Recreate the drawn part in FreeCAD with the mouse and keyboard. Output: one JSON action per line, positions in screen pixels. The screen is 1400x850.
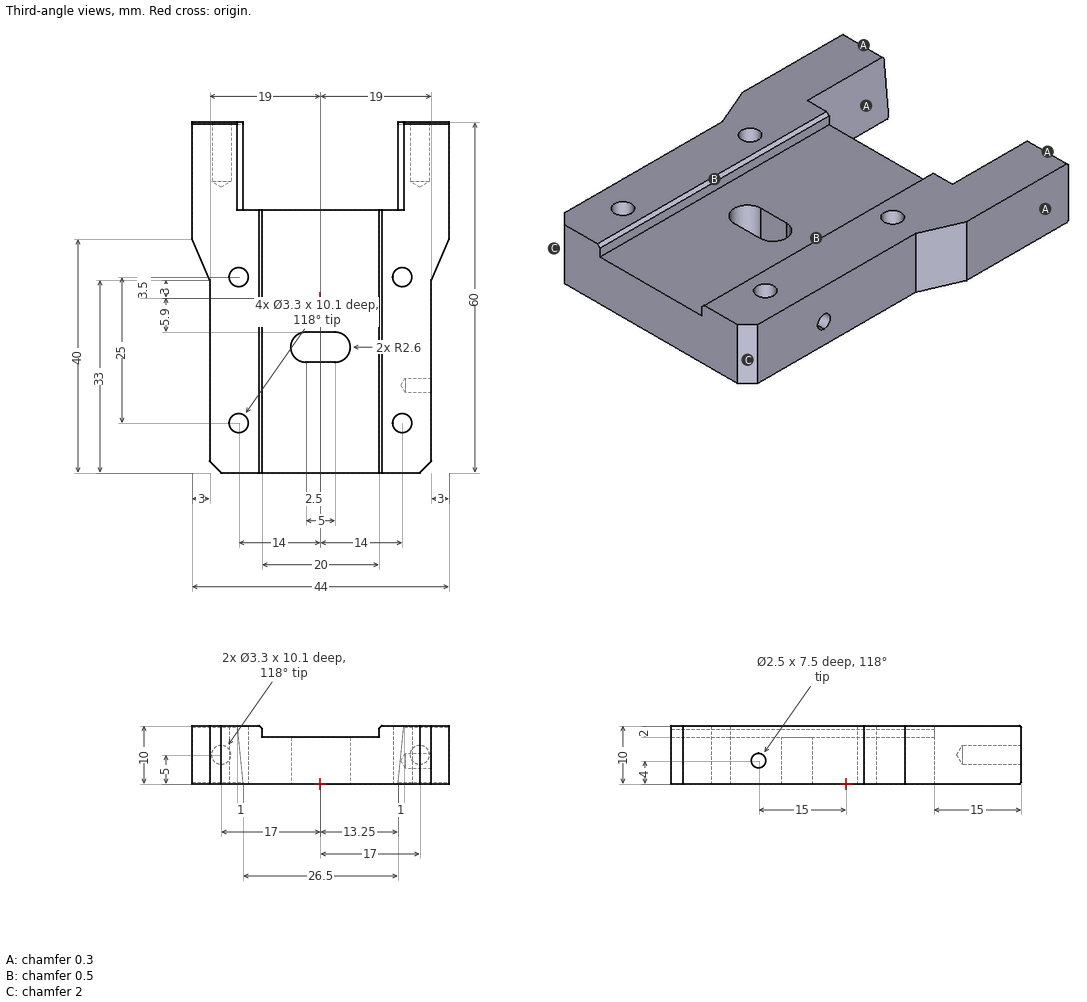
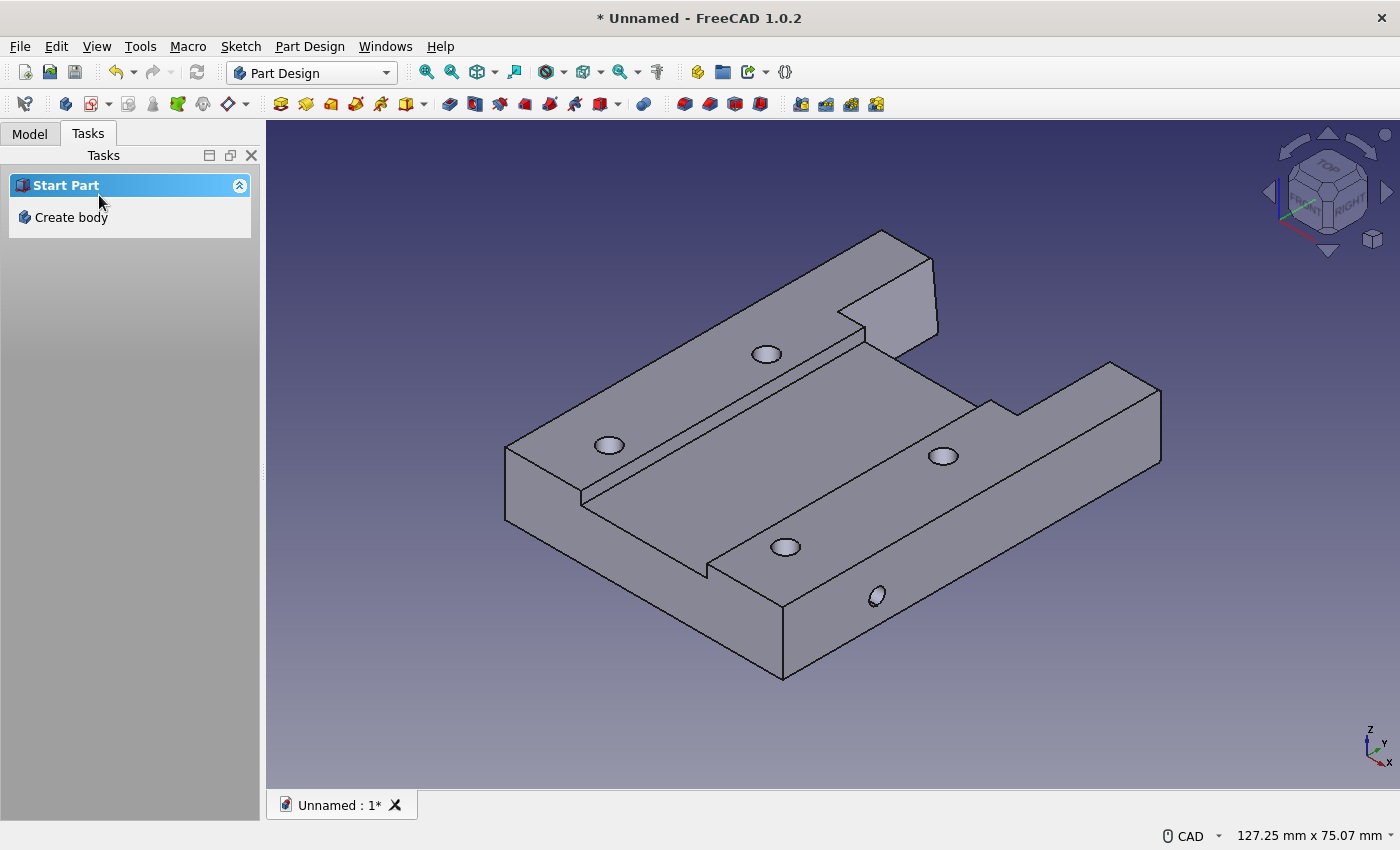
{"action": "left_click", "coordinate": [723, 408]}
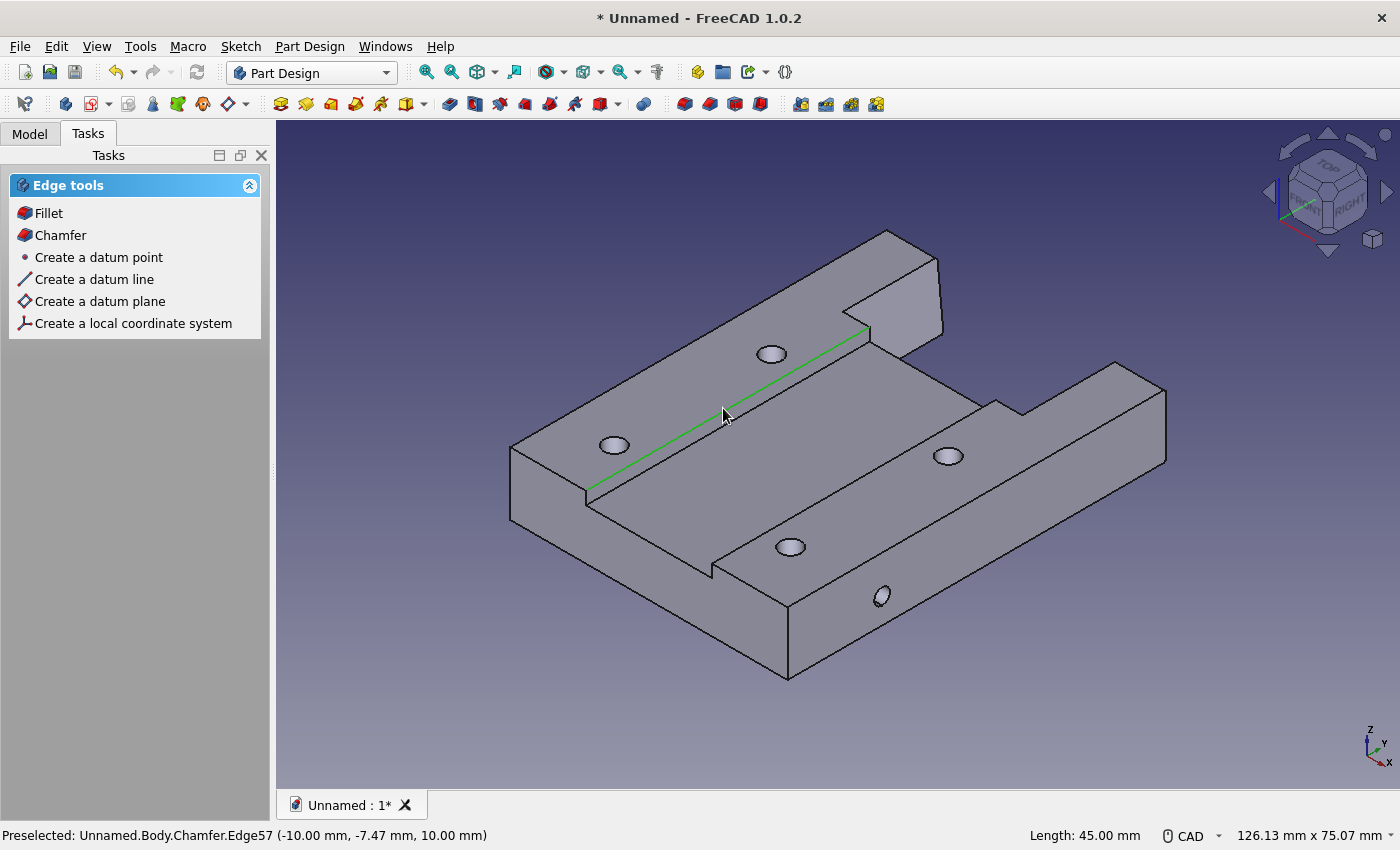
{"action": "key", "text": "2"}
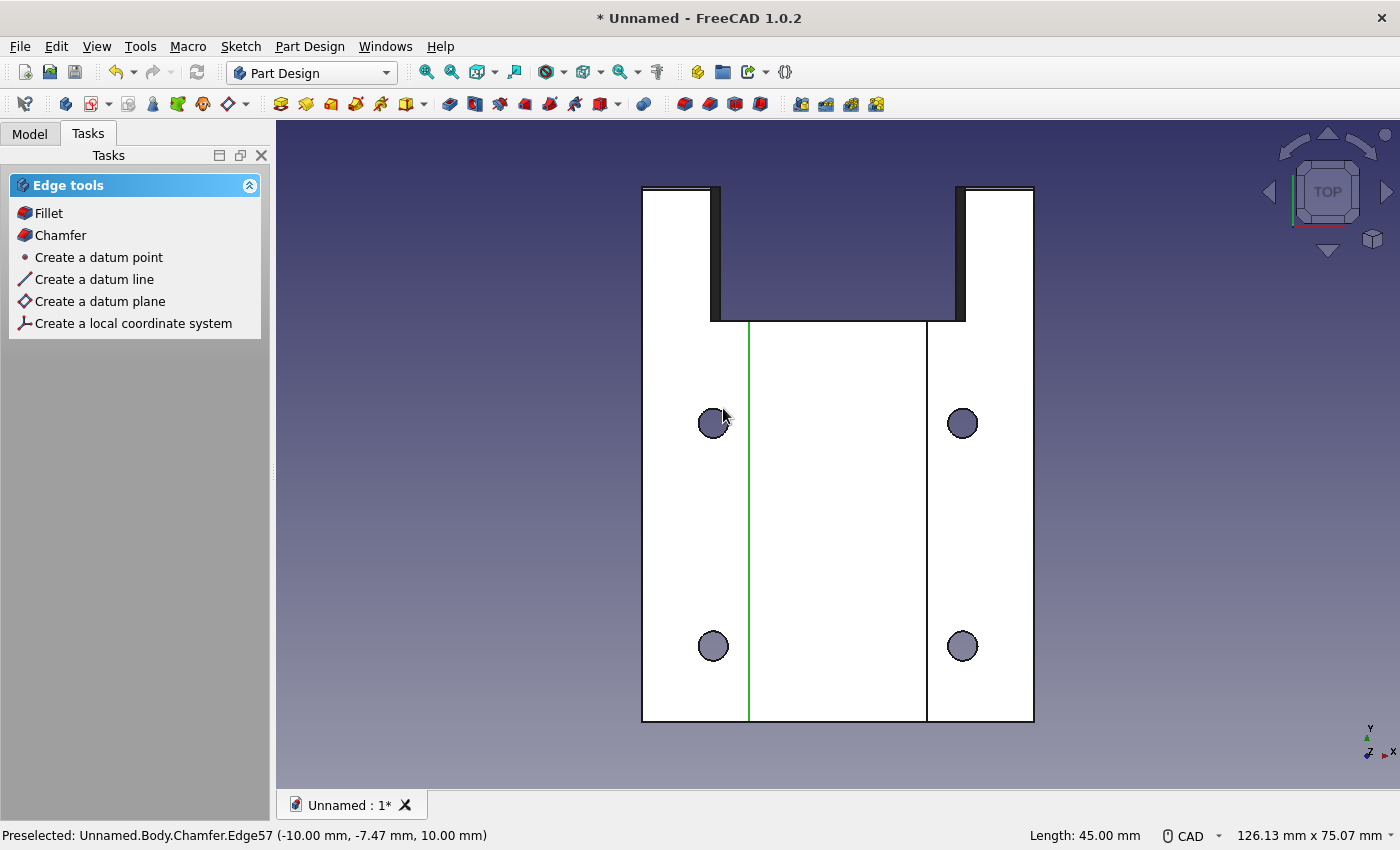
{"action": "left_click", "coordinate": [927, 520], "text": "ctrl"}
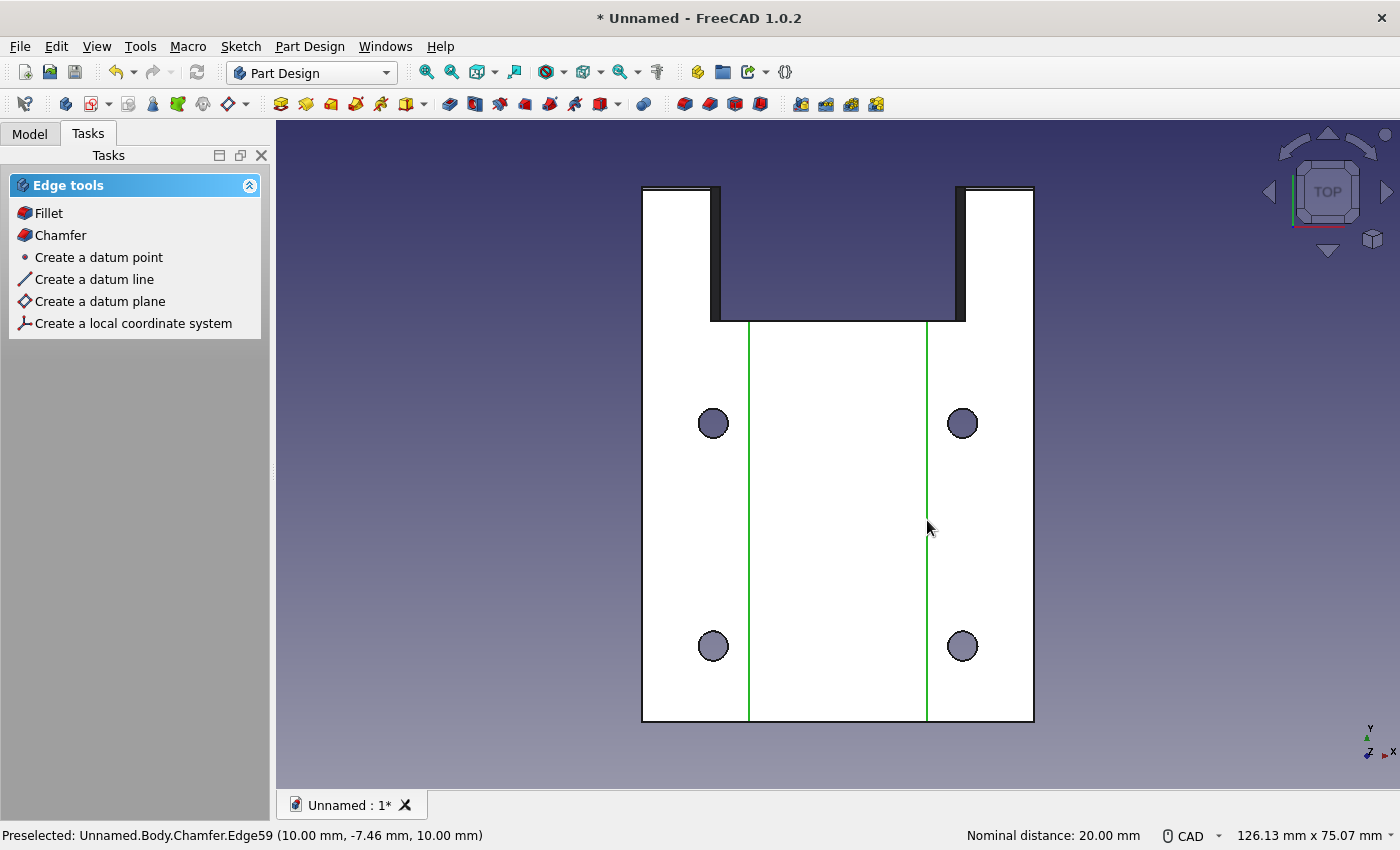
{"action": "left_click", "coordinate": [710, 104]}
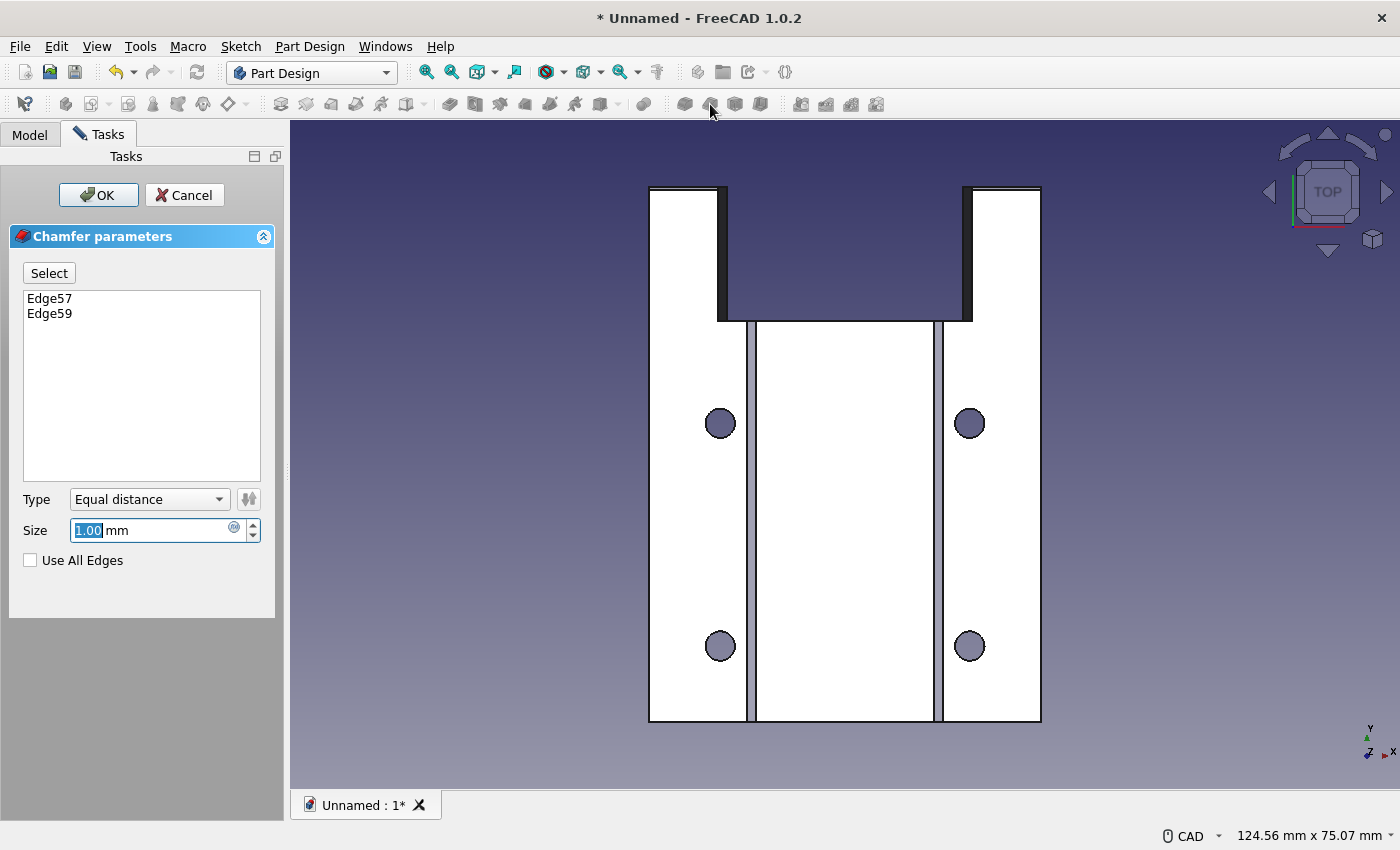
{"action": "type", "text": "0.5"}
{"action": "key", "text": "Tab"}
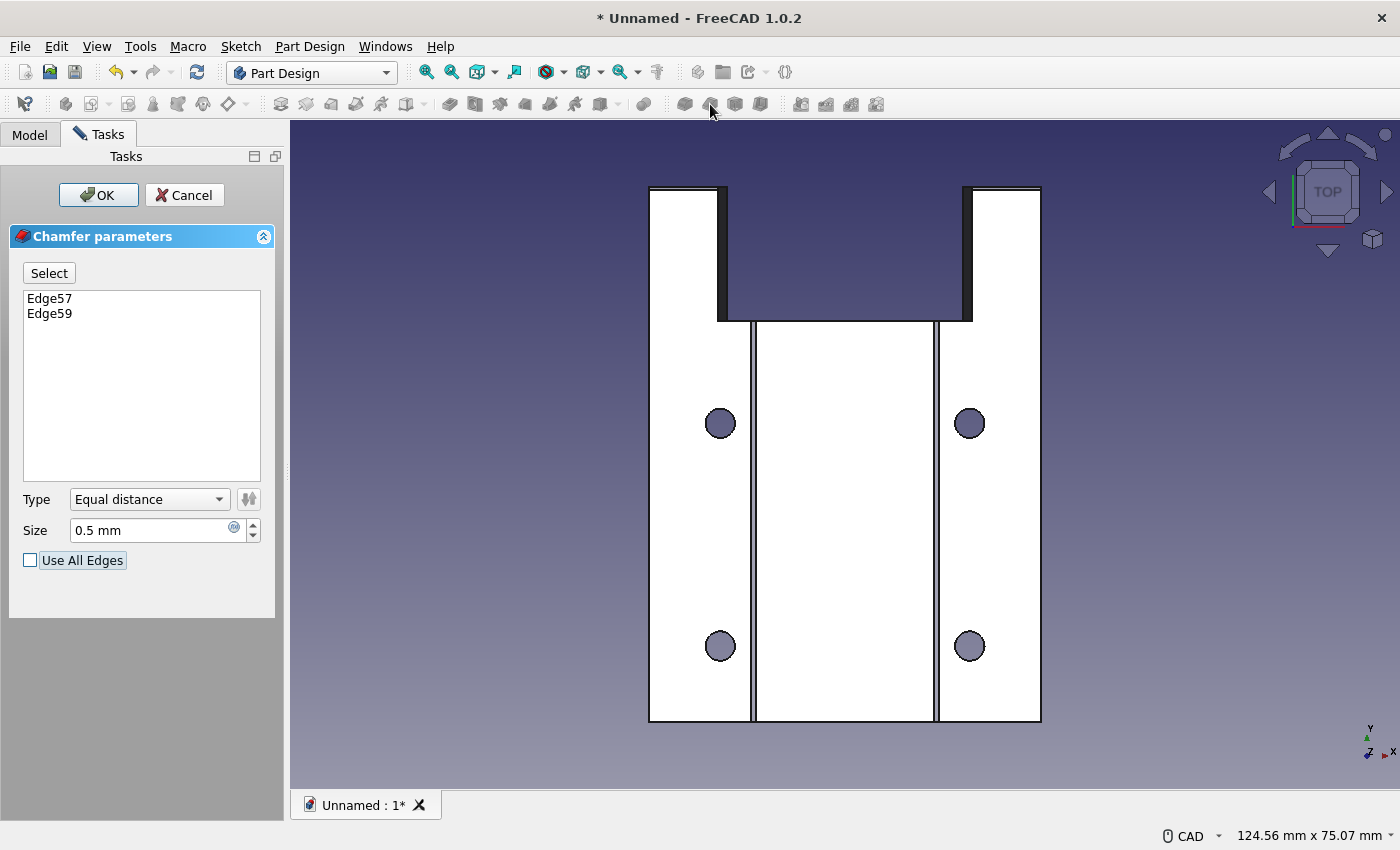
{"action": "left_click", "coordinate": [99, 195]}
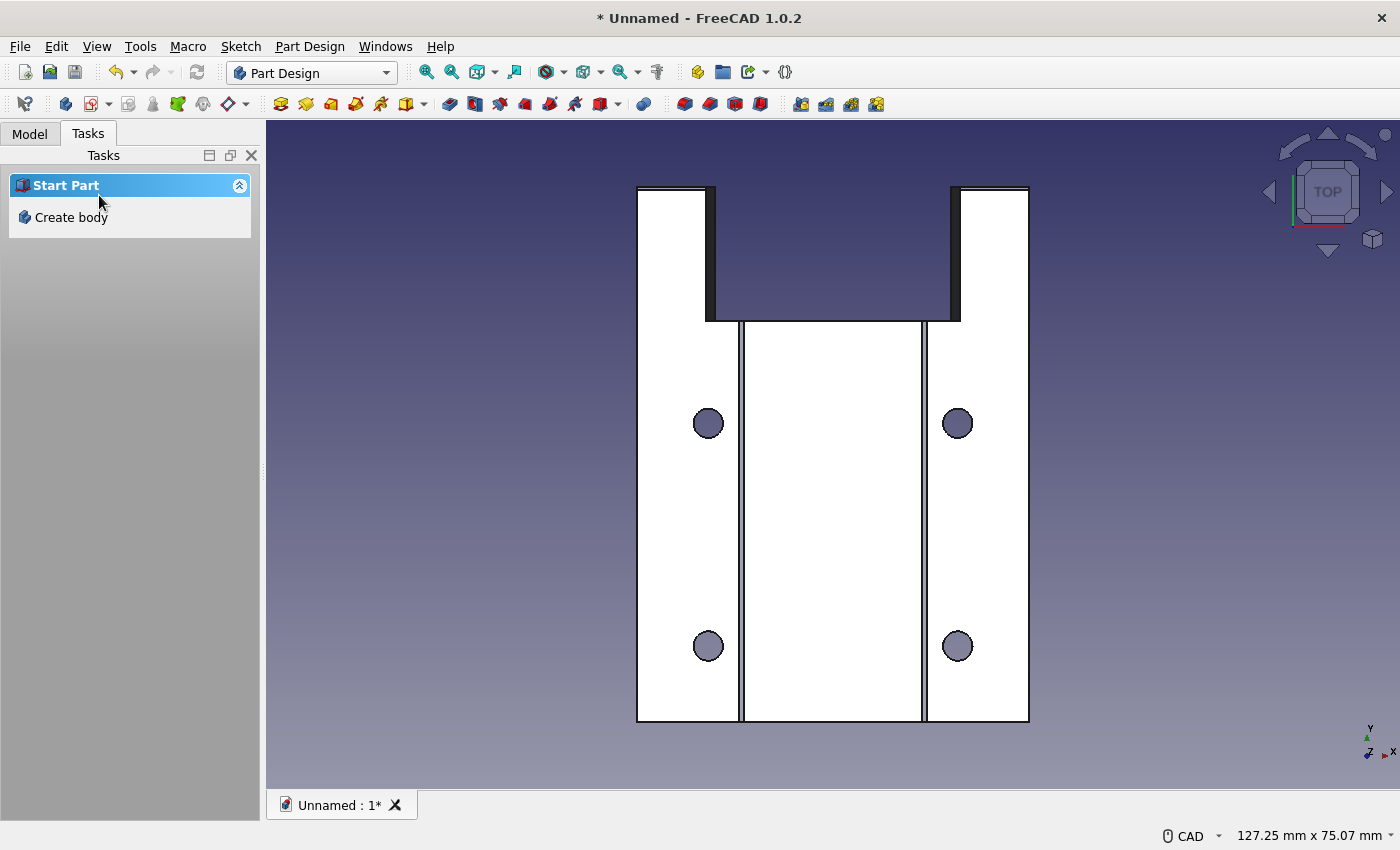
{"action": "left_click", "coordinate": [978, 531]}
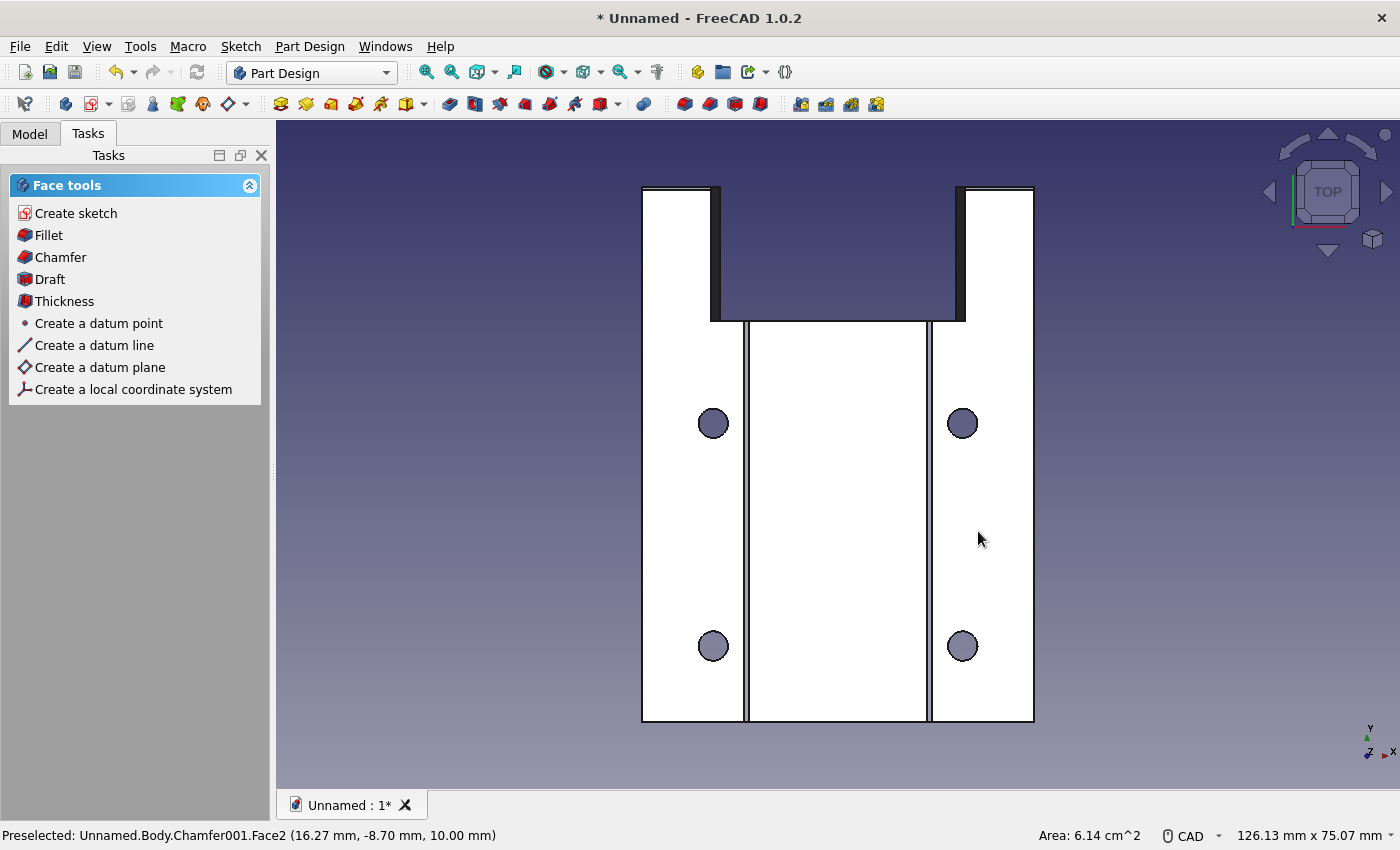
{"action": "left_click", "coordinate": [90, 104]}